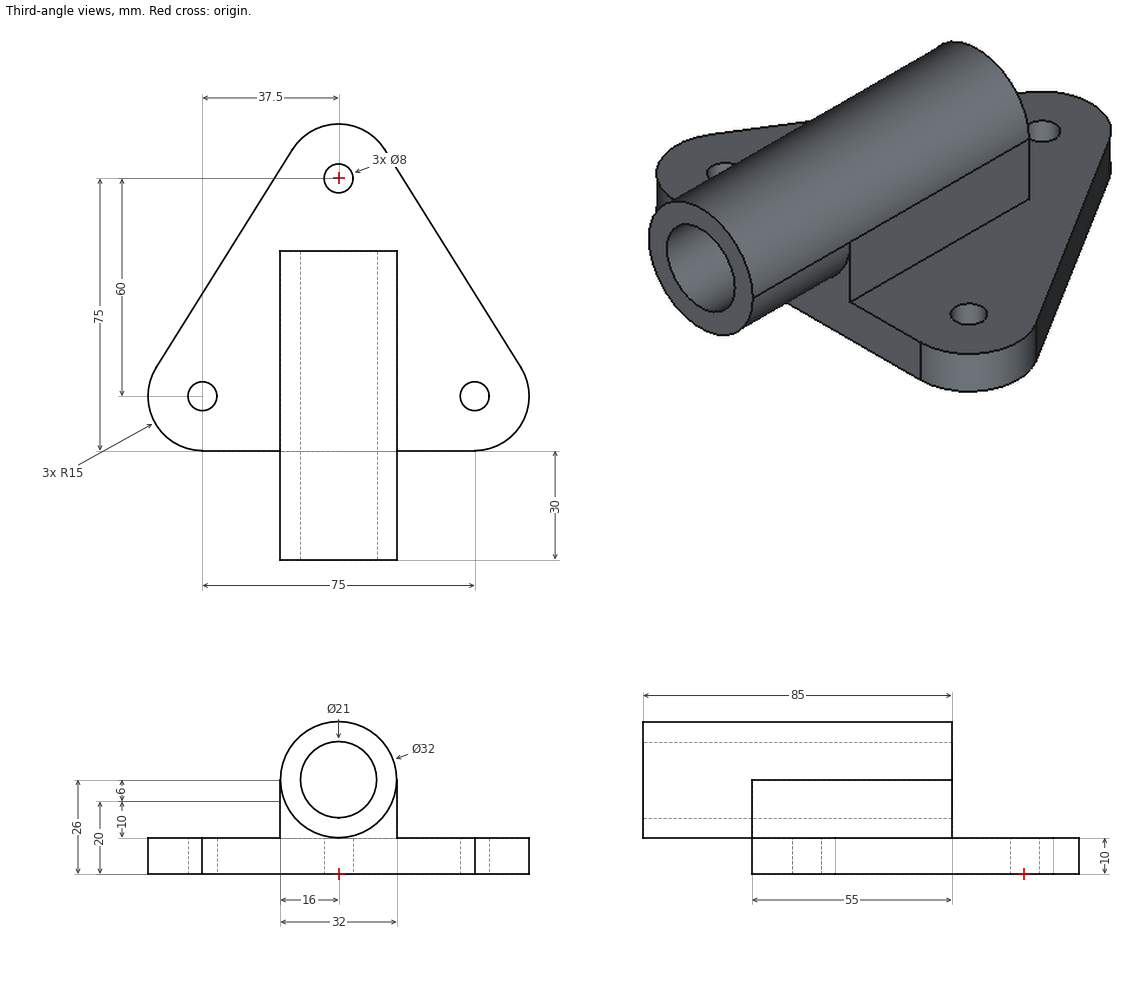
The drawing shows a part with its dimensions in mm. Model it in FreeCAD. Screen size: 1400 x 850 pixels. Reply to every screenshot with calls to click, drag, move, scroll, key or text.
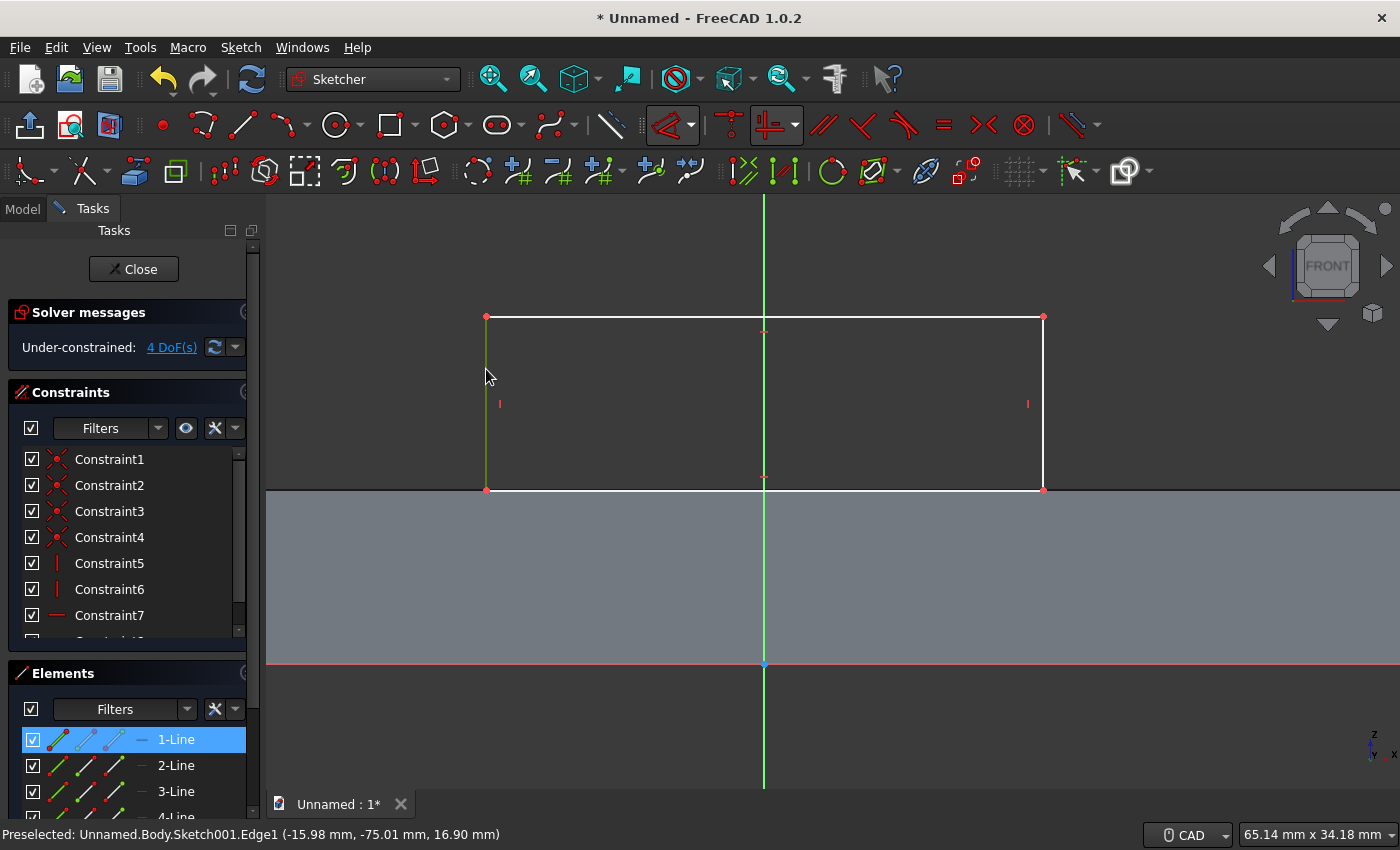
click(694, 126)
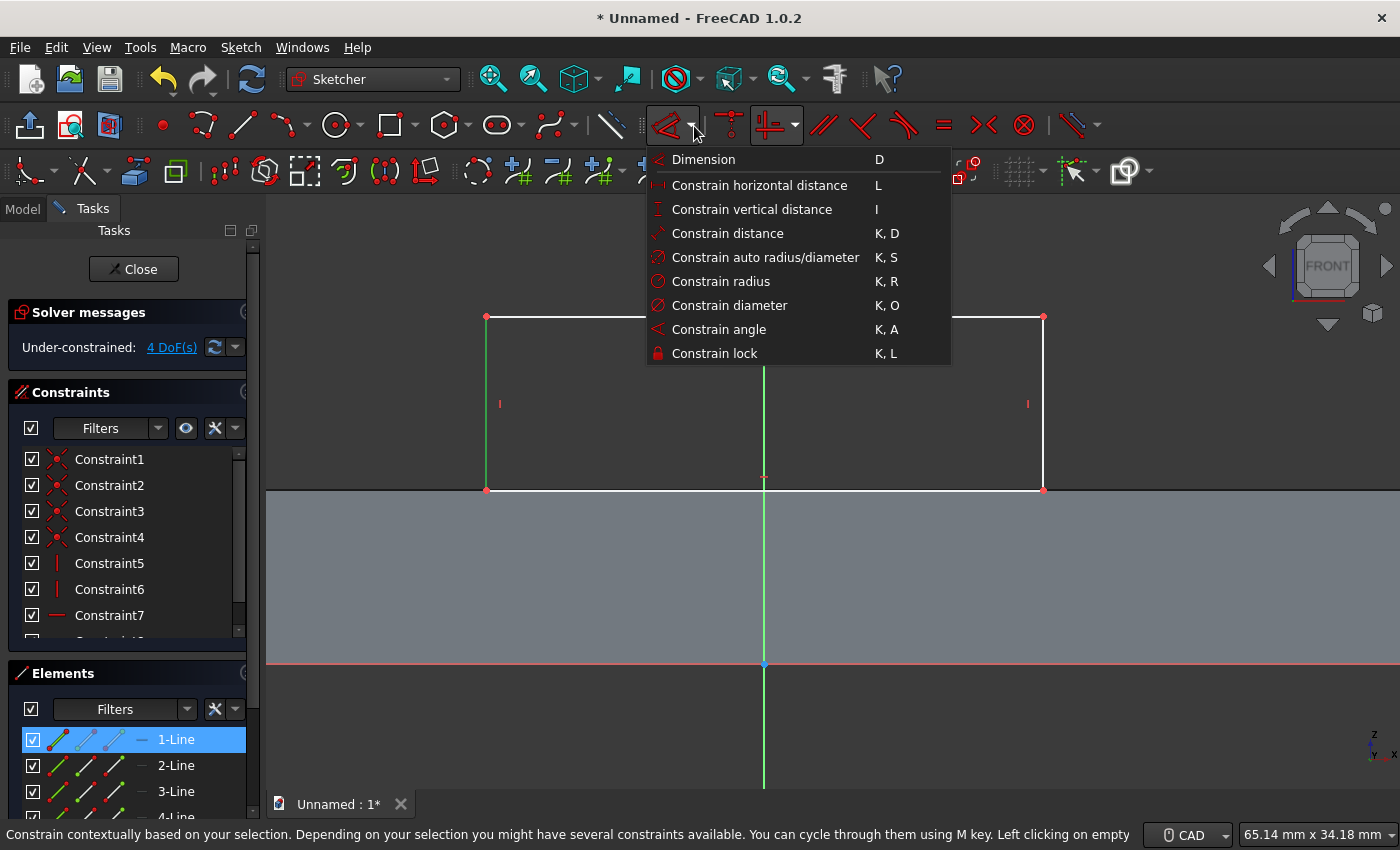
click(799, 209)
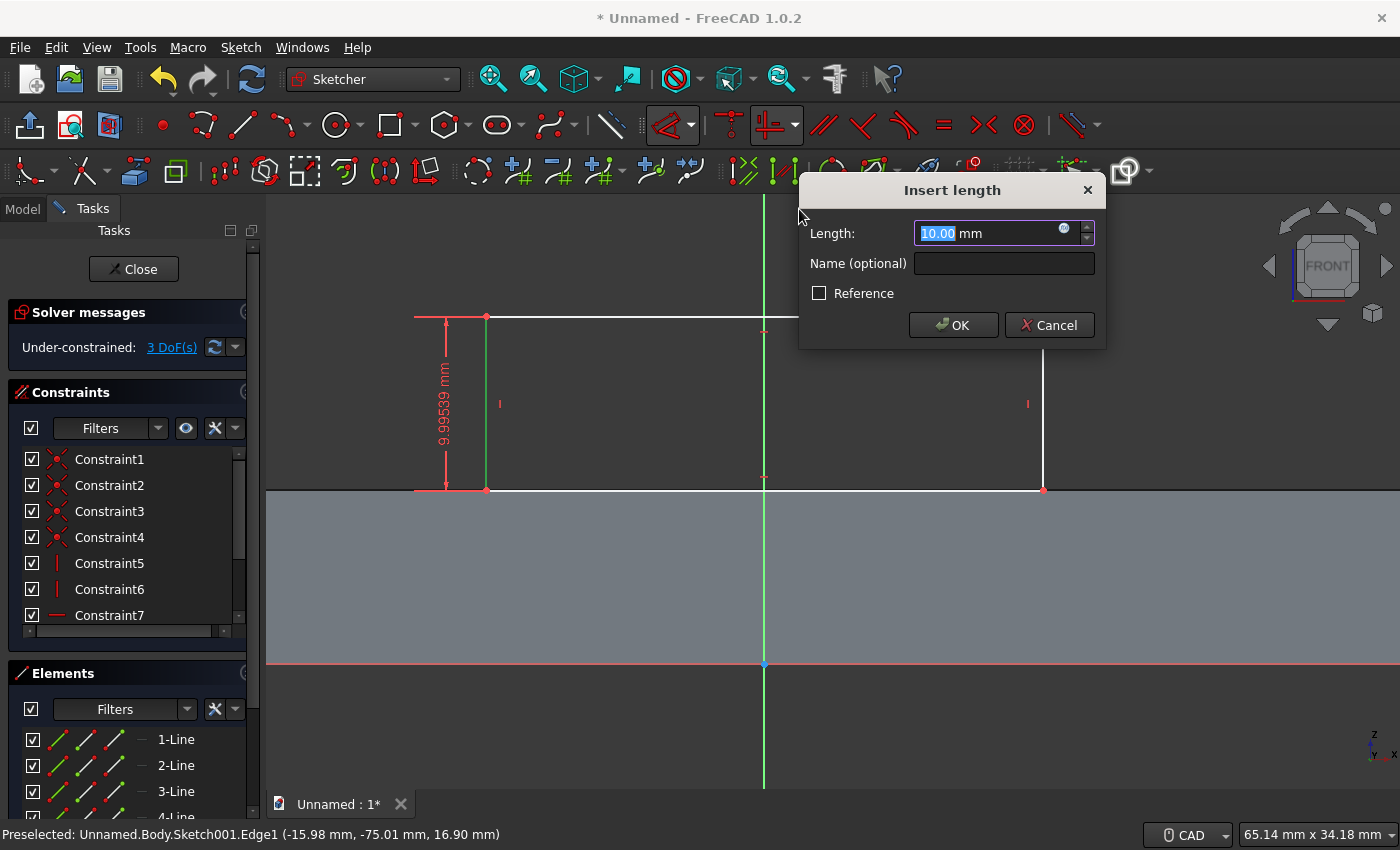
text(10)
key(Return)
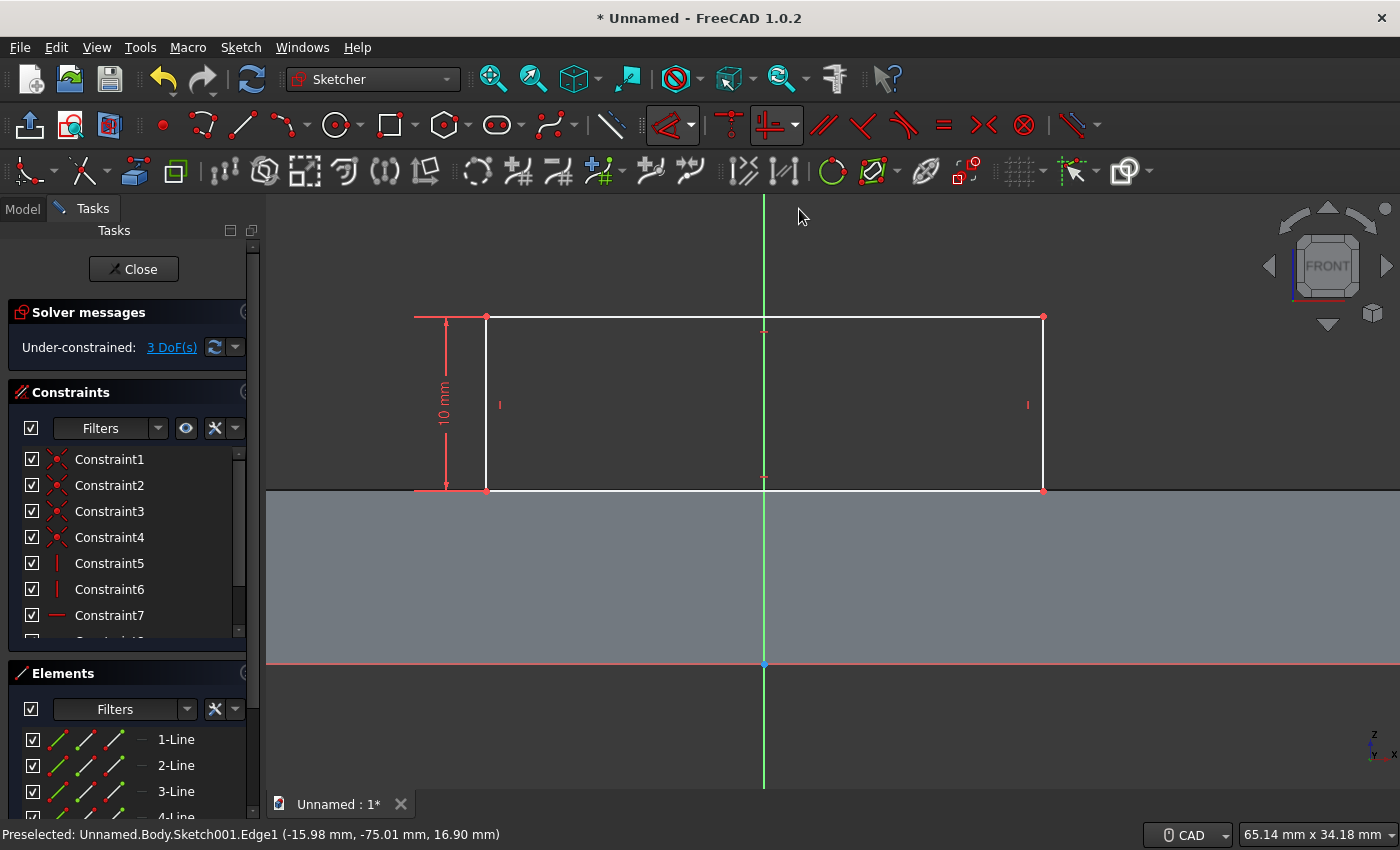
click(653, 491)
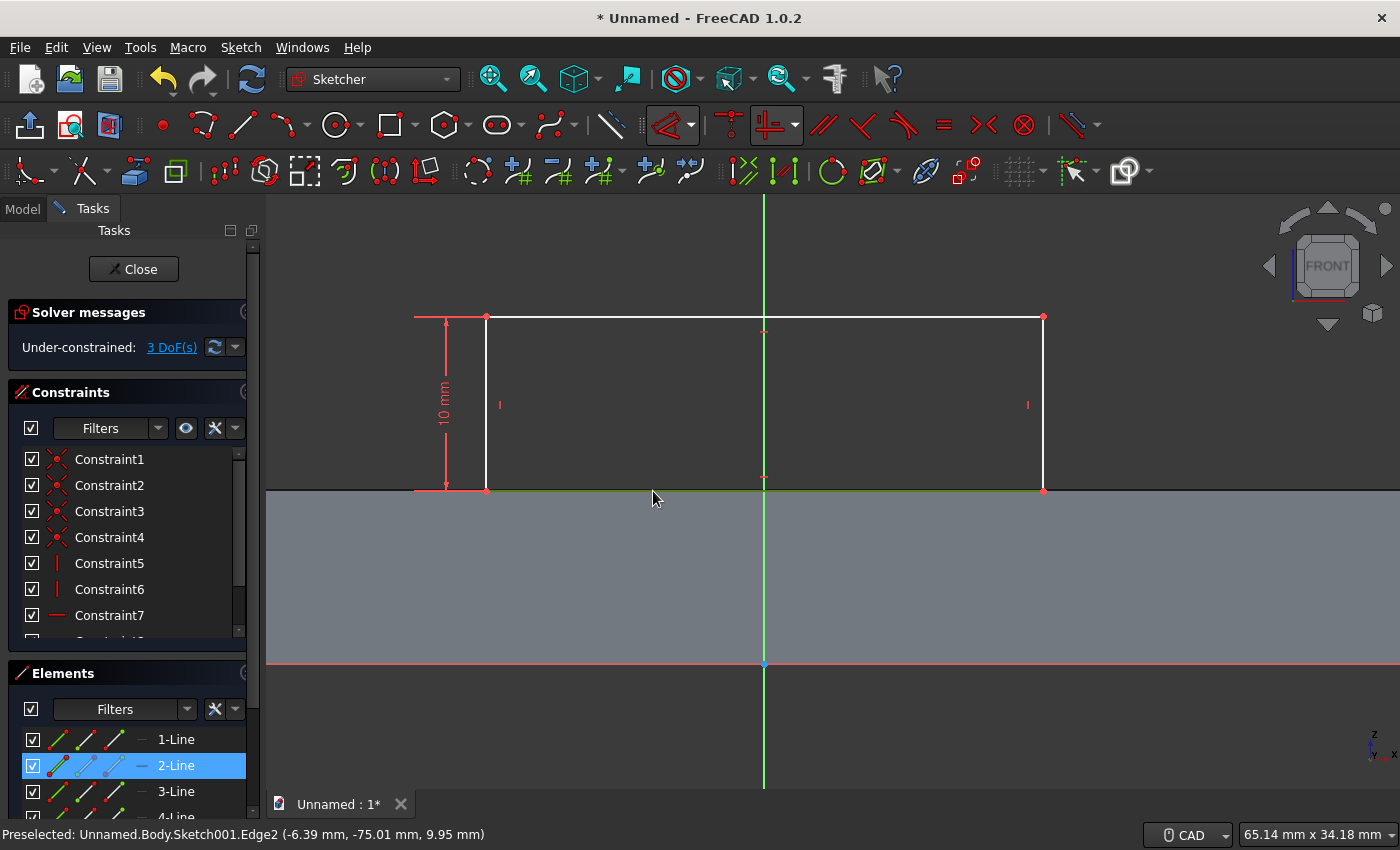
key(l)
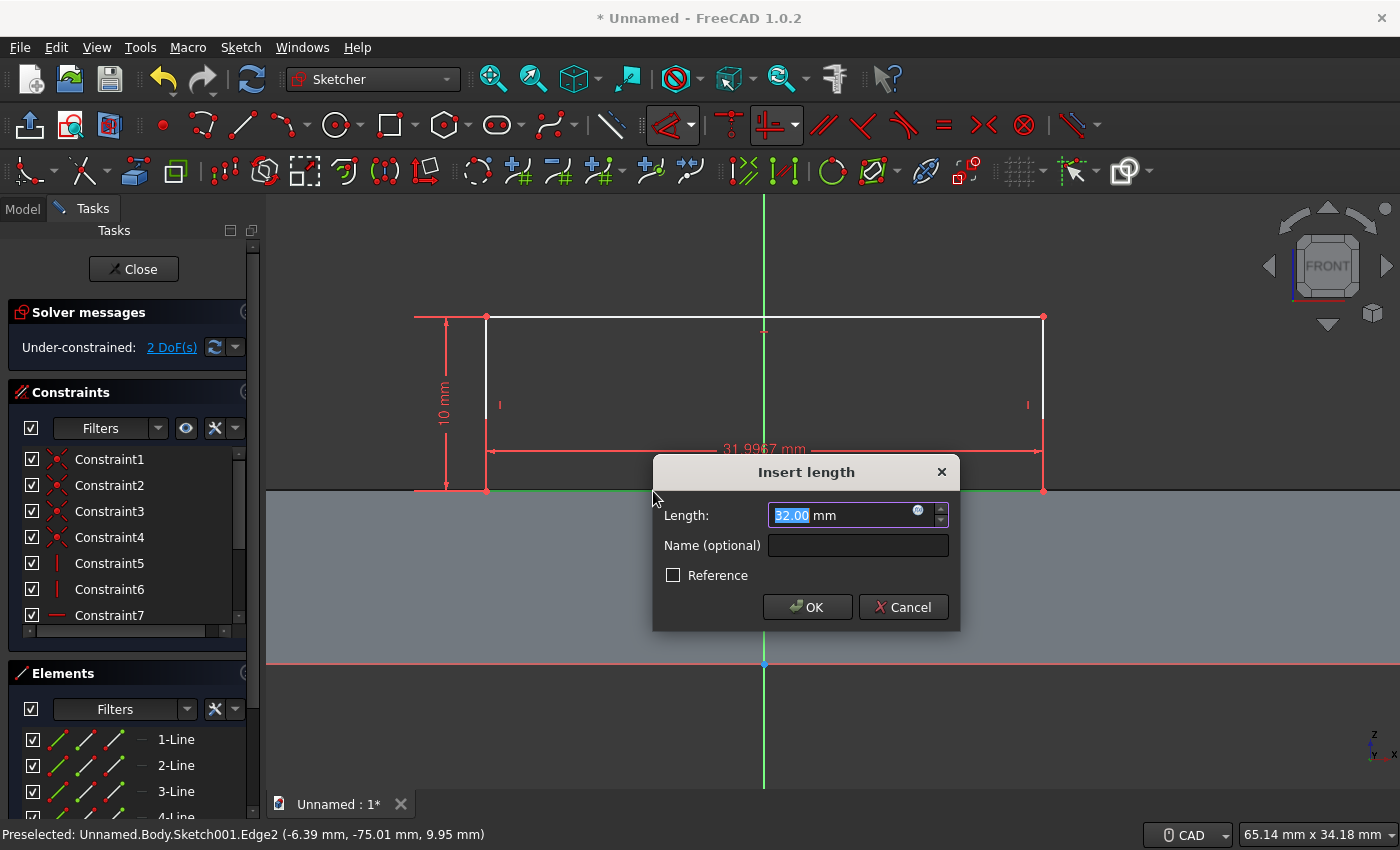
text(32)
key(Return)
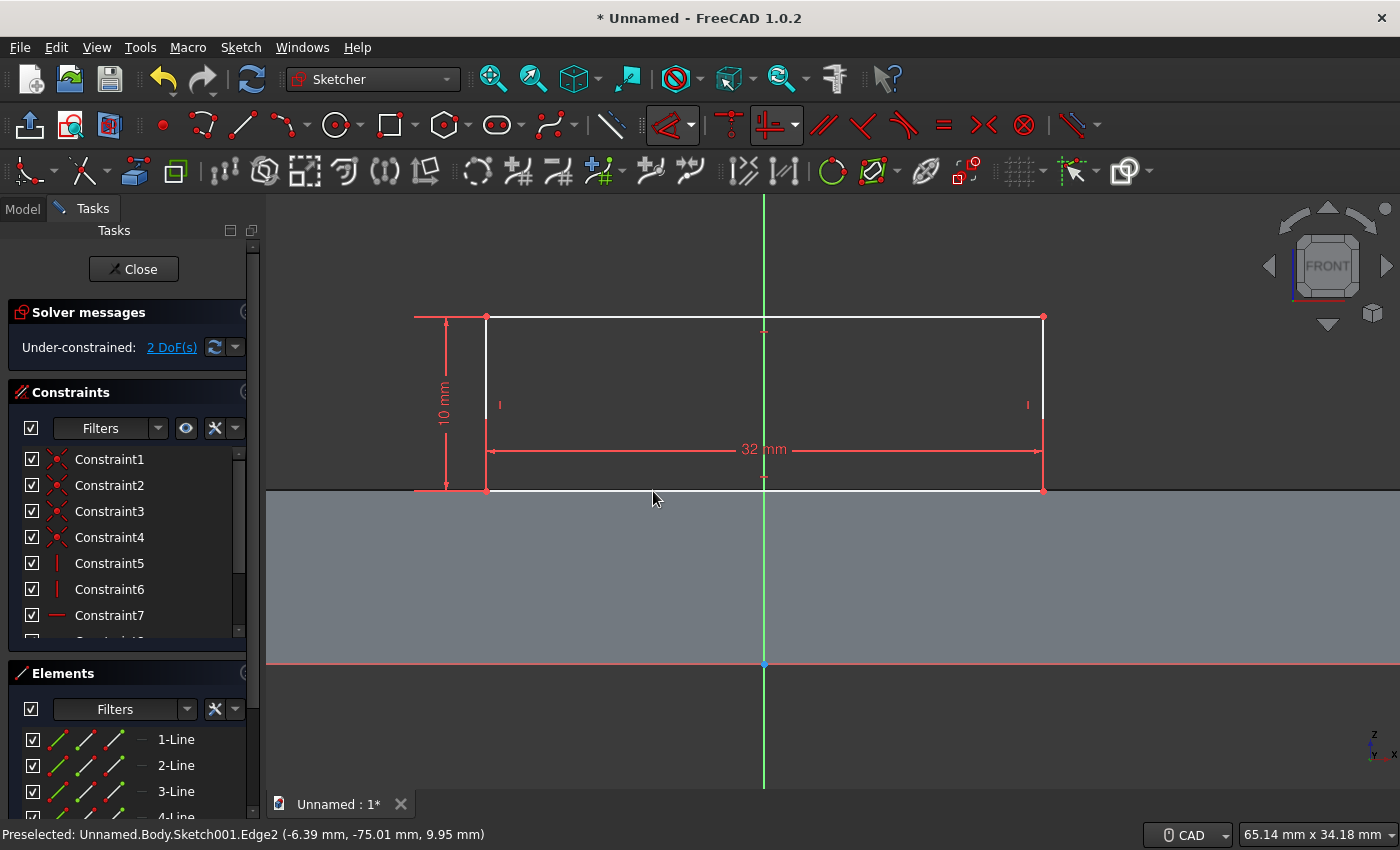
click(486, 317)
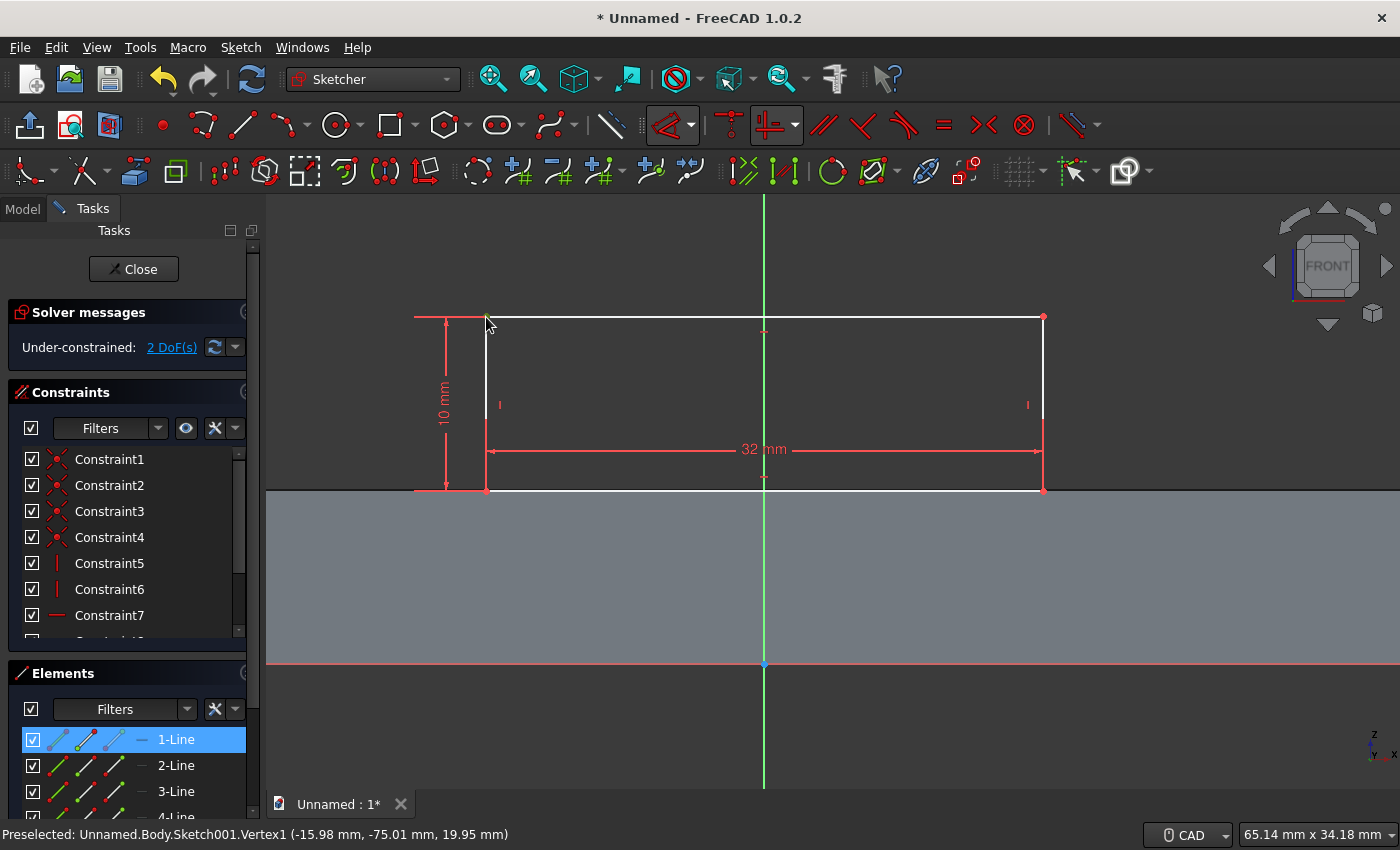
key(l)